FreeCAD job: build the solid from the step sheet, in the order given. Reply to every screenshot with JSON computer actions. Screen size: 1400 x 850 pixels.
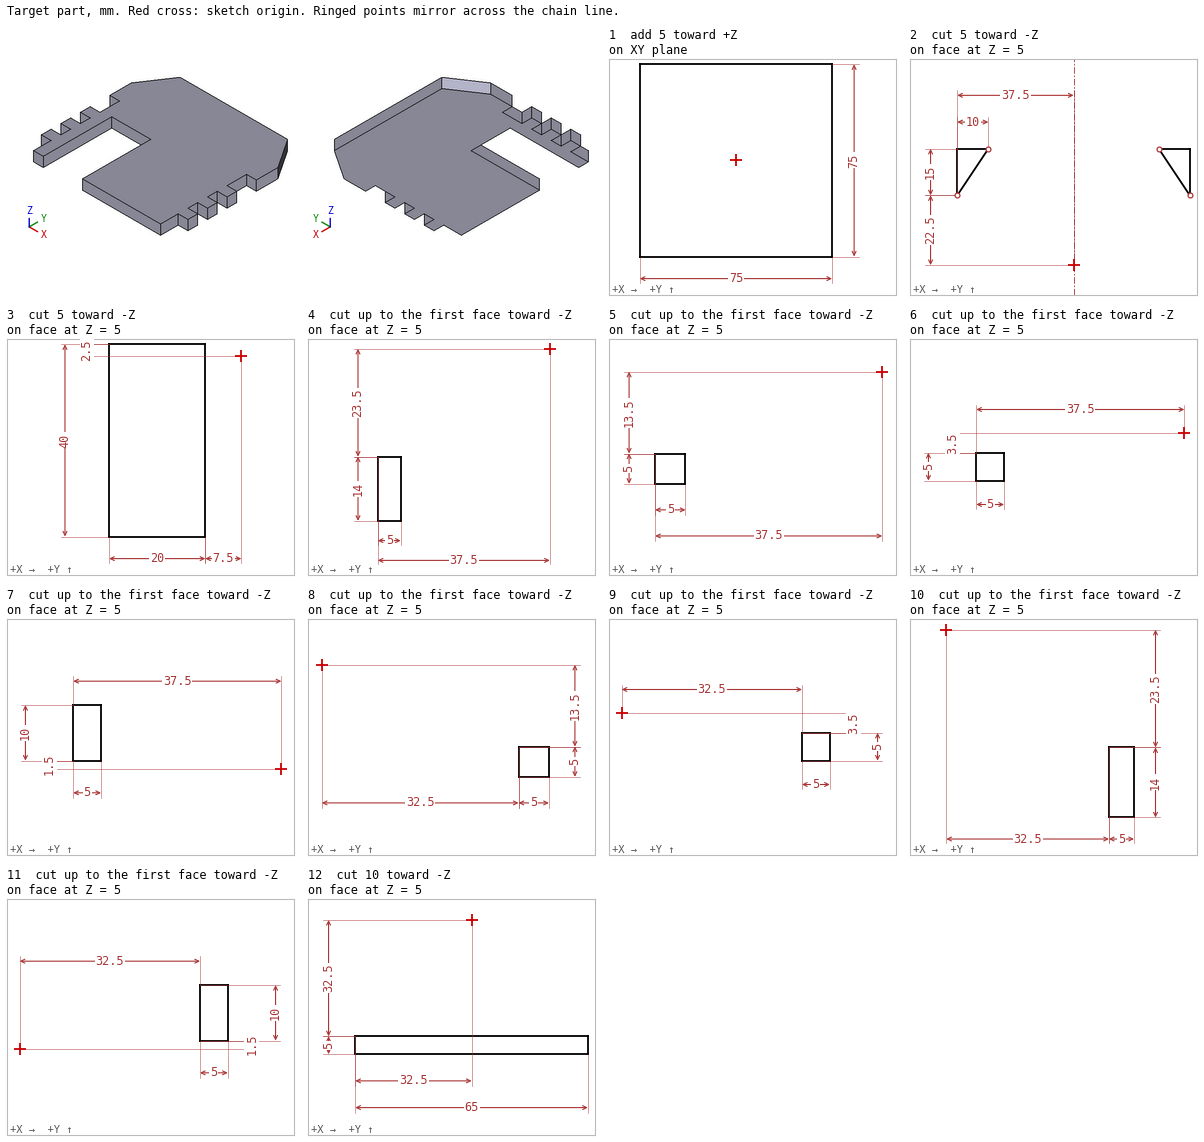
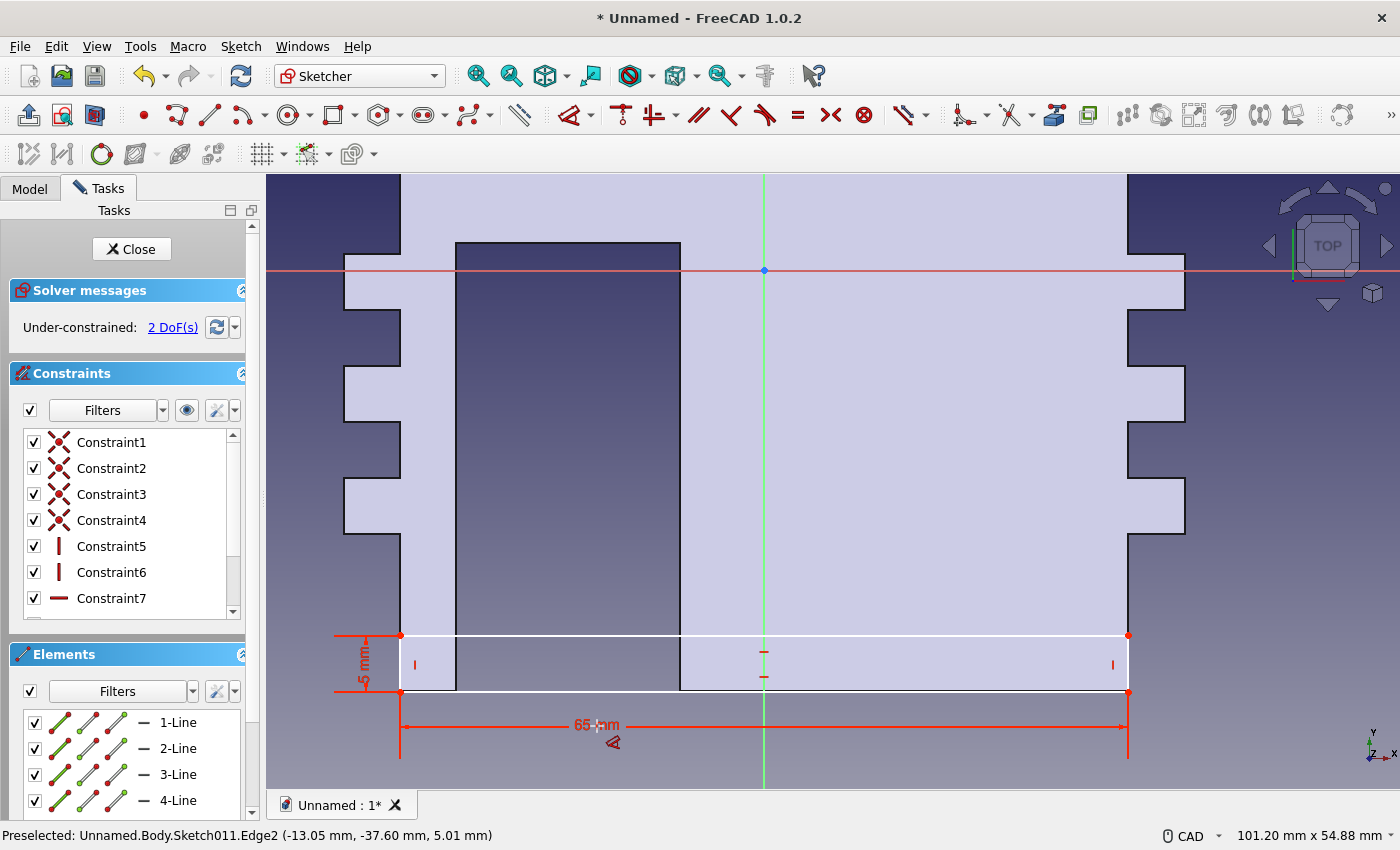
{"action": "left_click", "coordinate": [400, 636]}
{"action": "left_click", "coordinate": [582, 237]}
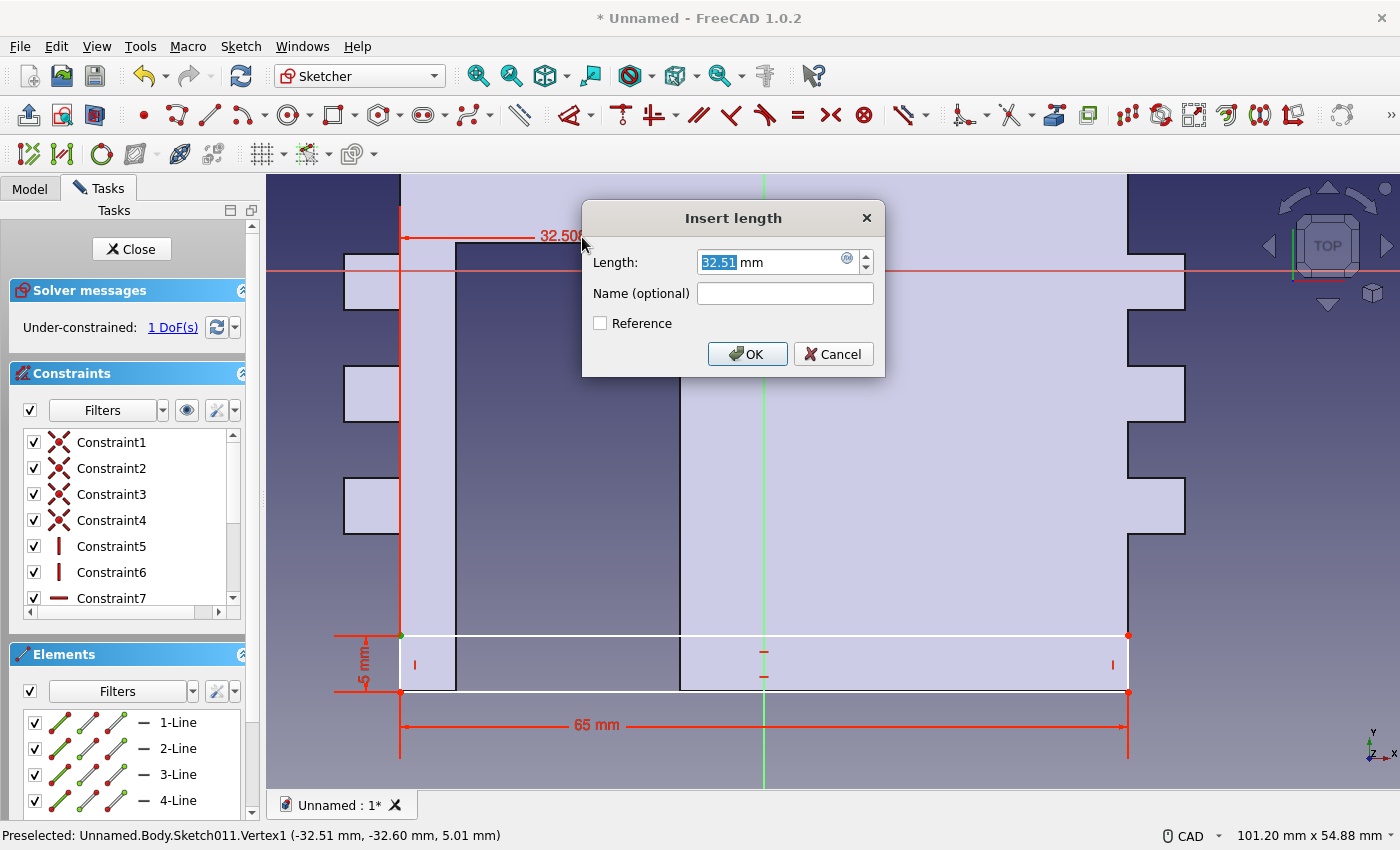
{"action": "type", "text": "32.5"}
{"action": "key", "text": "Return"}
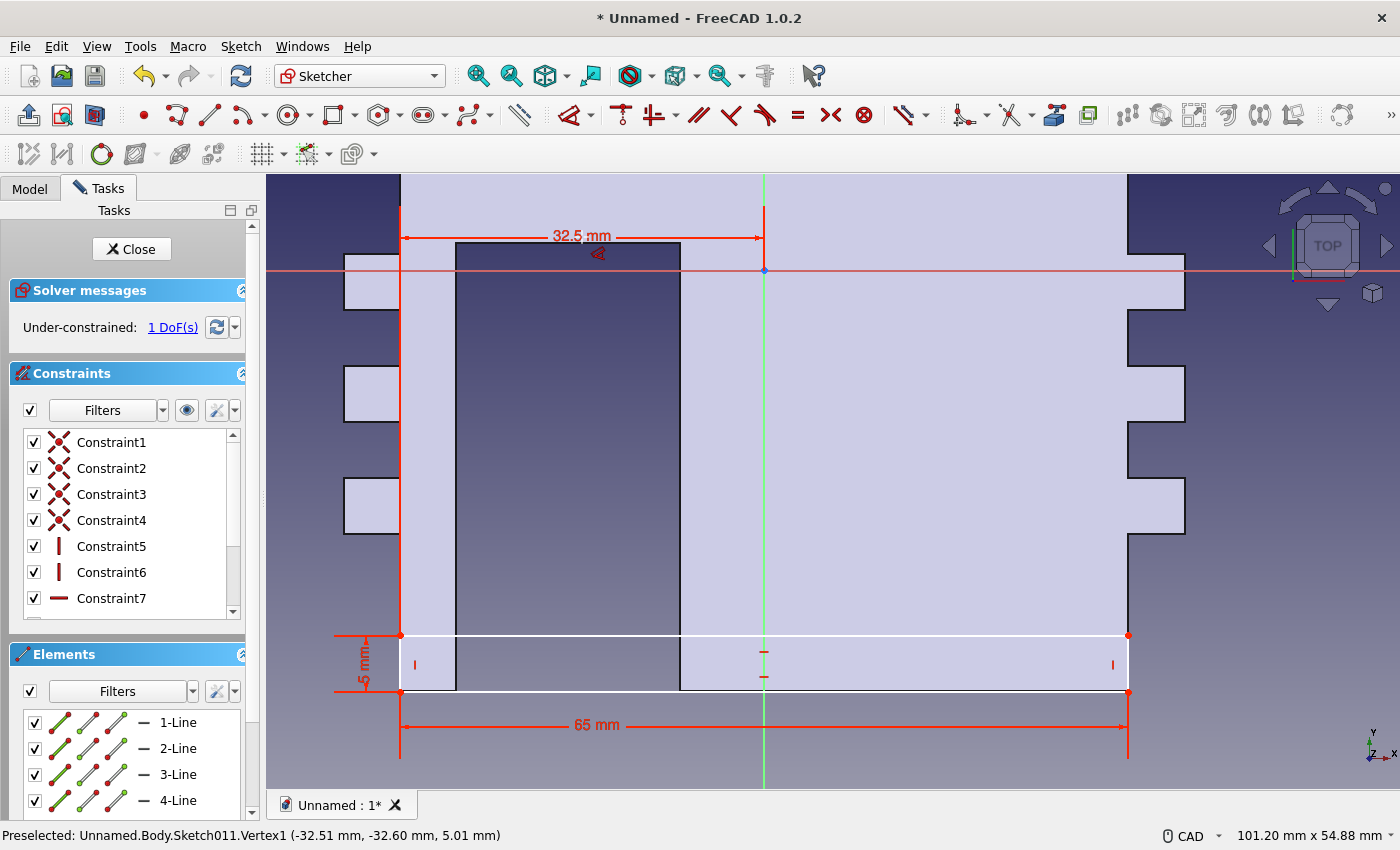
{"action": "left_click", "coordinate": [400, 636]}
{"action": "left_click", "coordinate": [366, 453]}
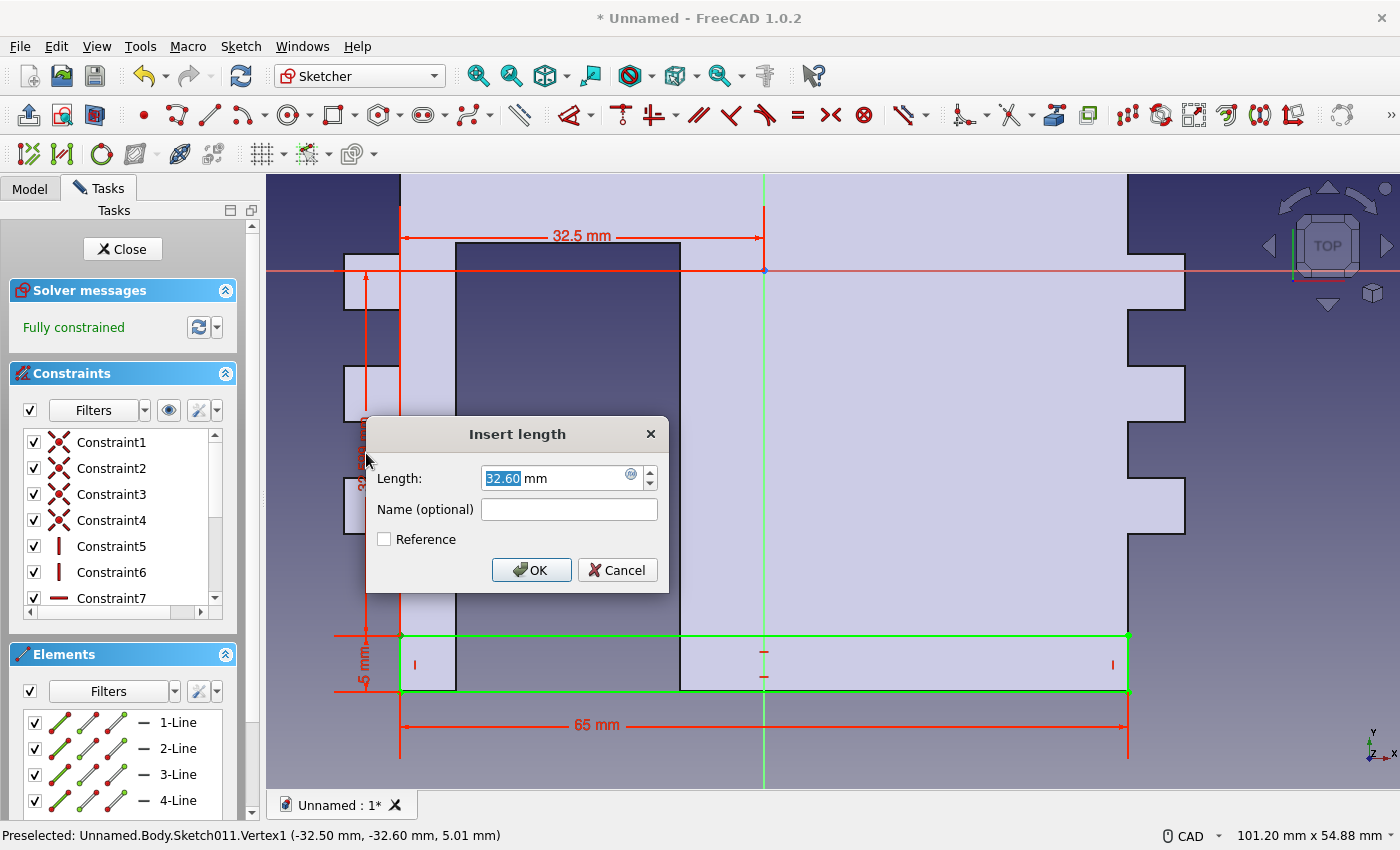
{"action": "type", "text": "32.5"}
{"action": "key", "text": "Return"}
{"action": "key", "text": "Escape"}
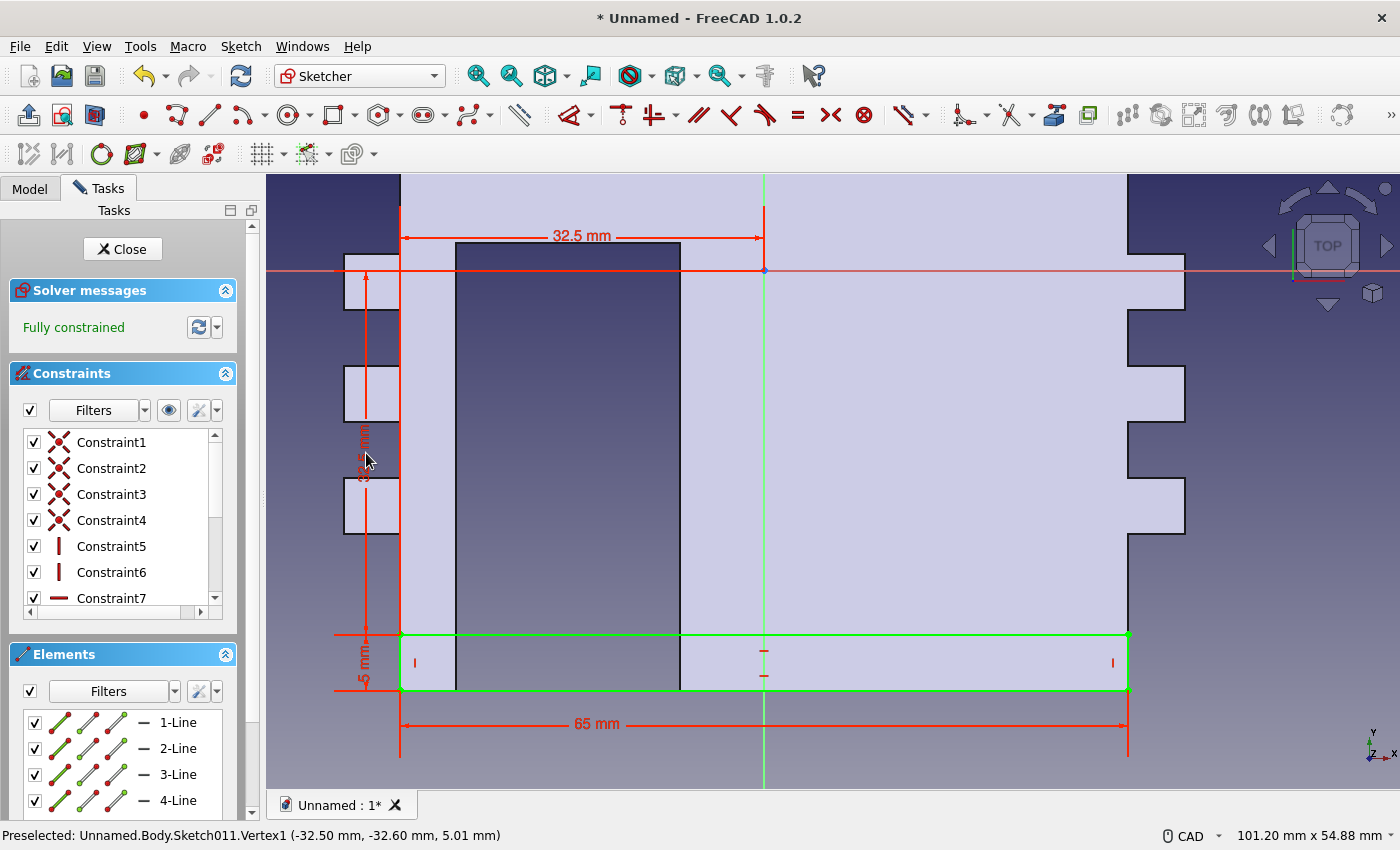
{"action": "left_click", "coordinate": [123, 249]}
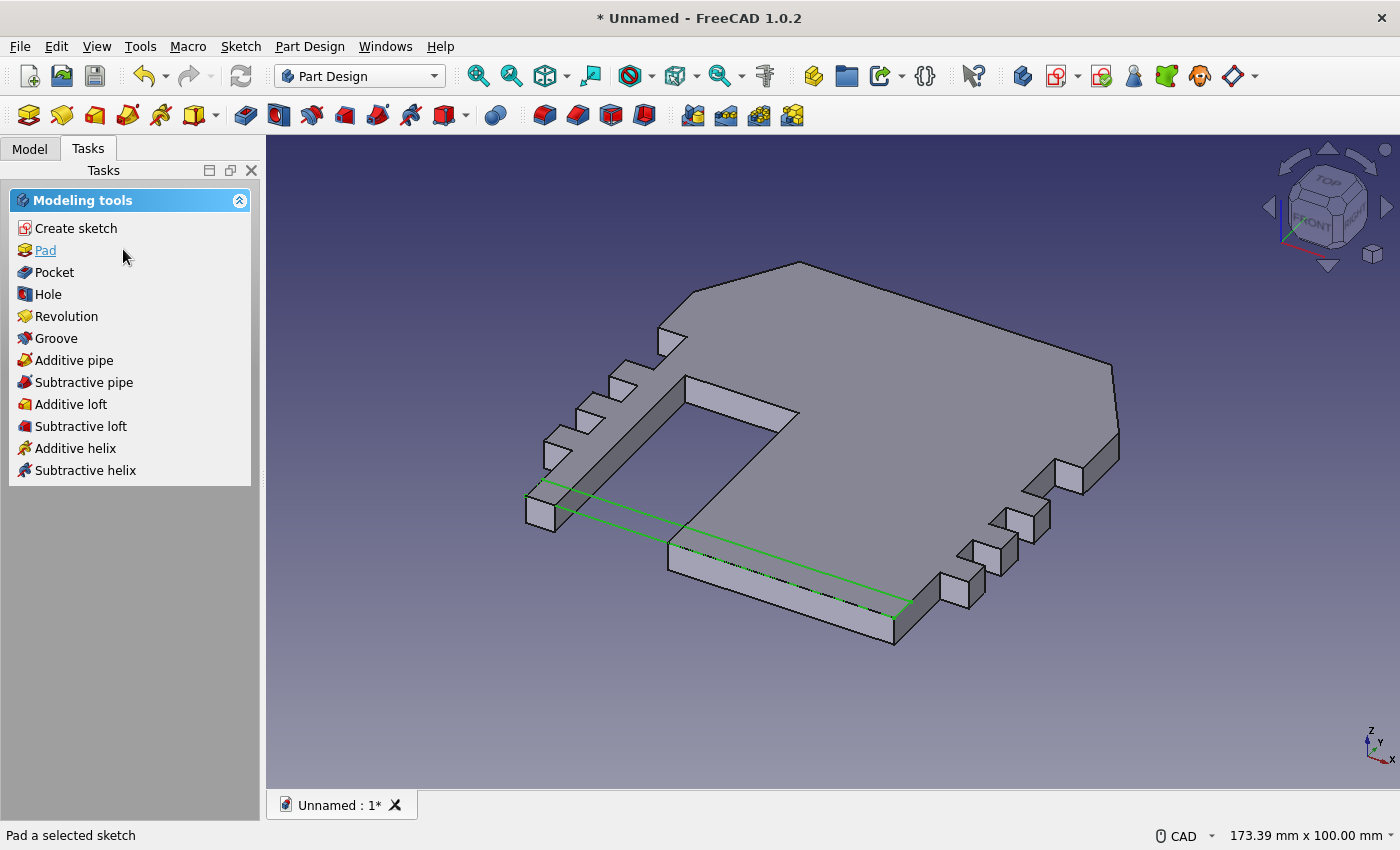
{"action": "left_click", "coordinate": [246, 116]}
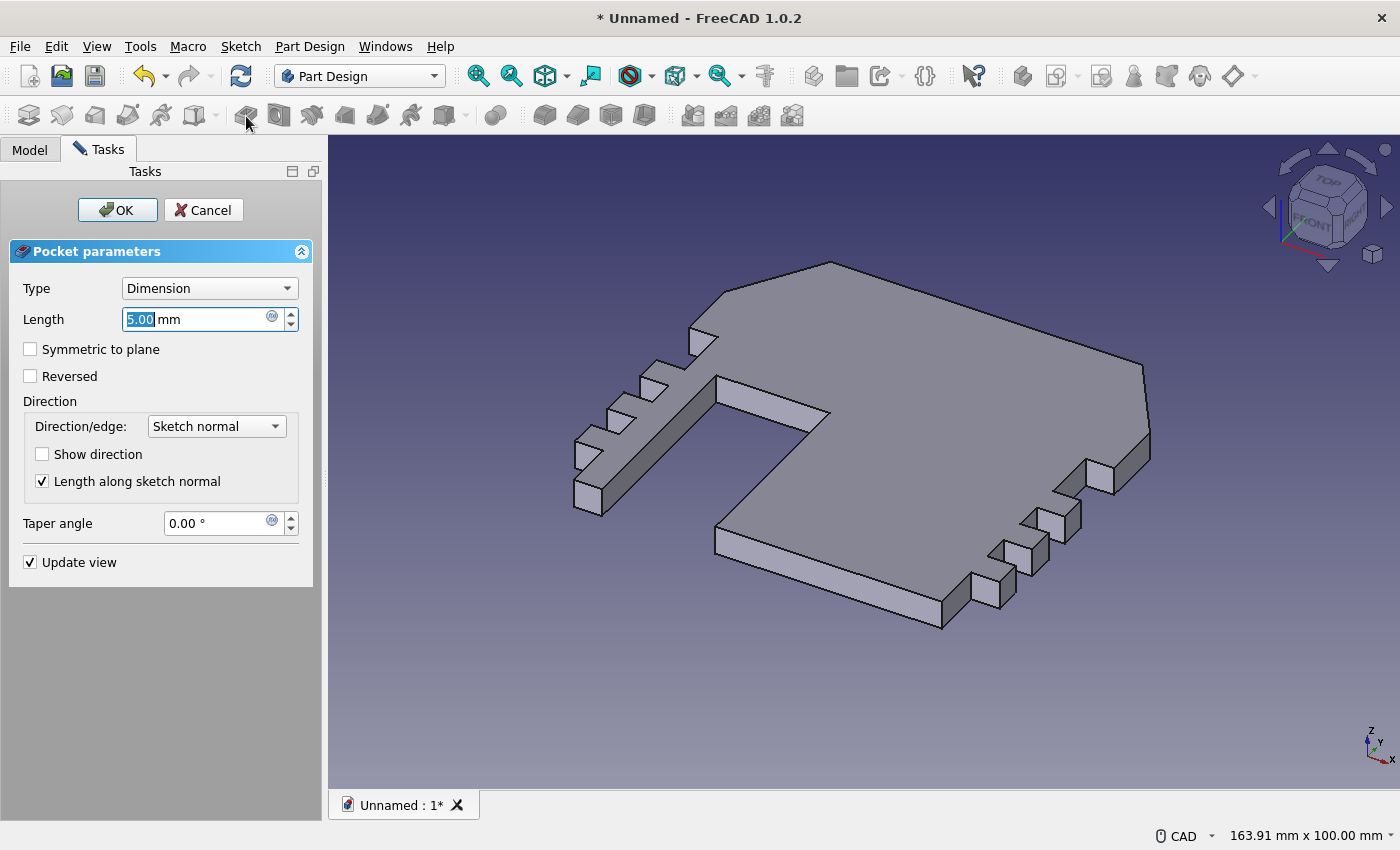
{"action": "type", "text": "10"}
{"action": "key", "text": "Tab"}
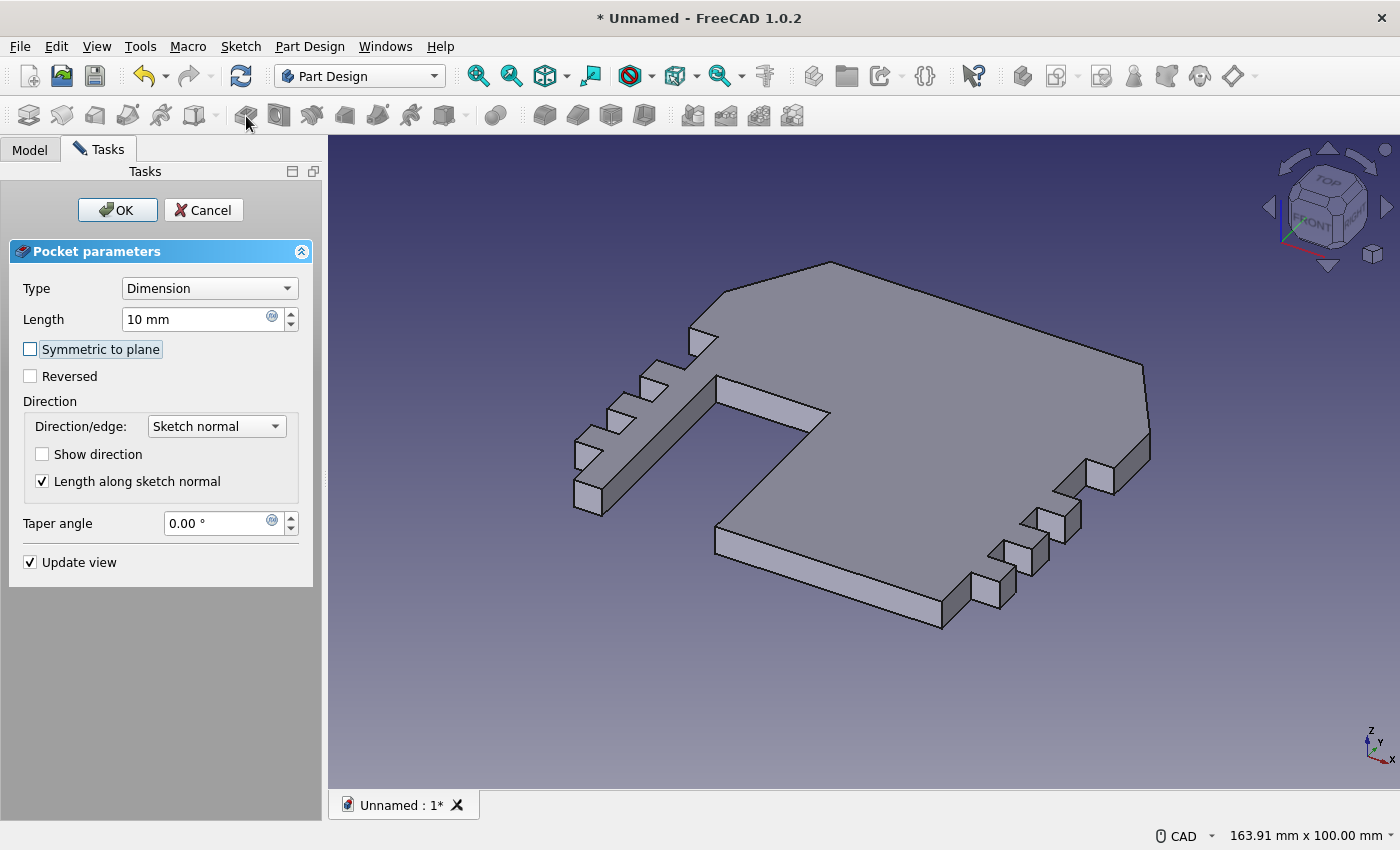
{"action": "left_click", "coordinate": [118, 210]}